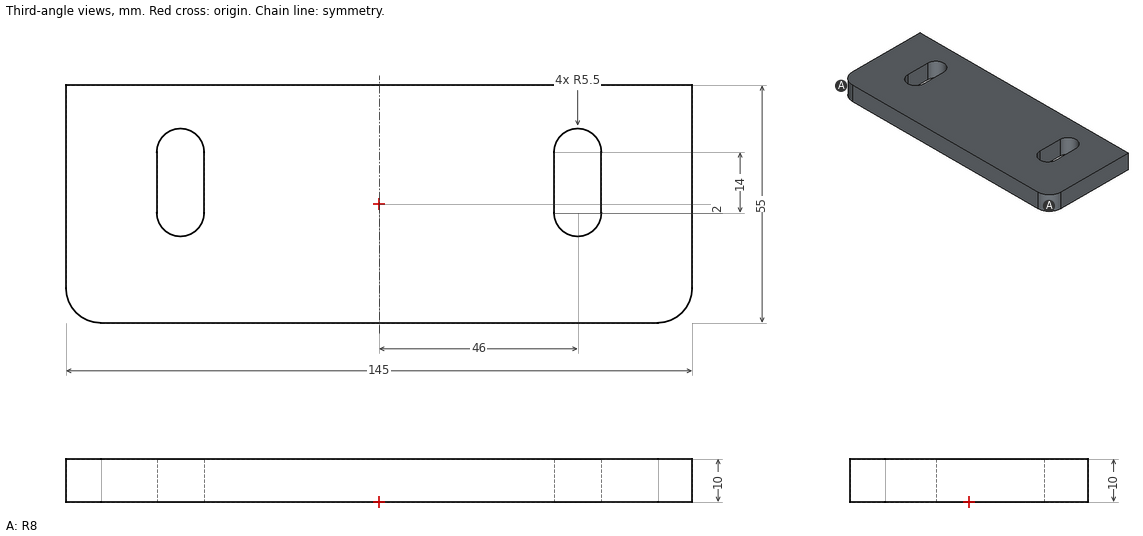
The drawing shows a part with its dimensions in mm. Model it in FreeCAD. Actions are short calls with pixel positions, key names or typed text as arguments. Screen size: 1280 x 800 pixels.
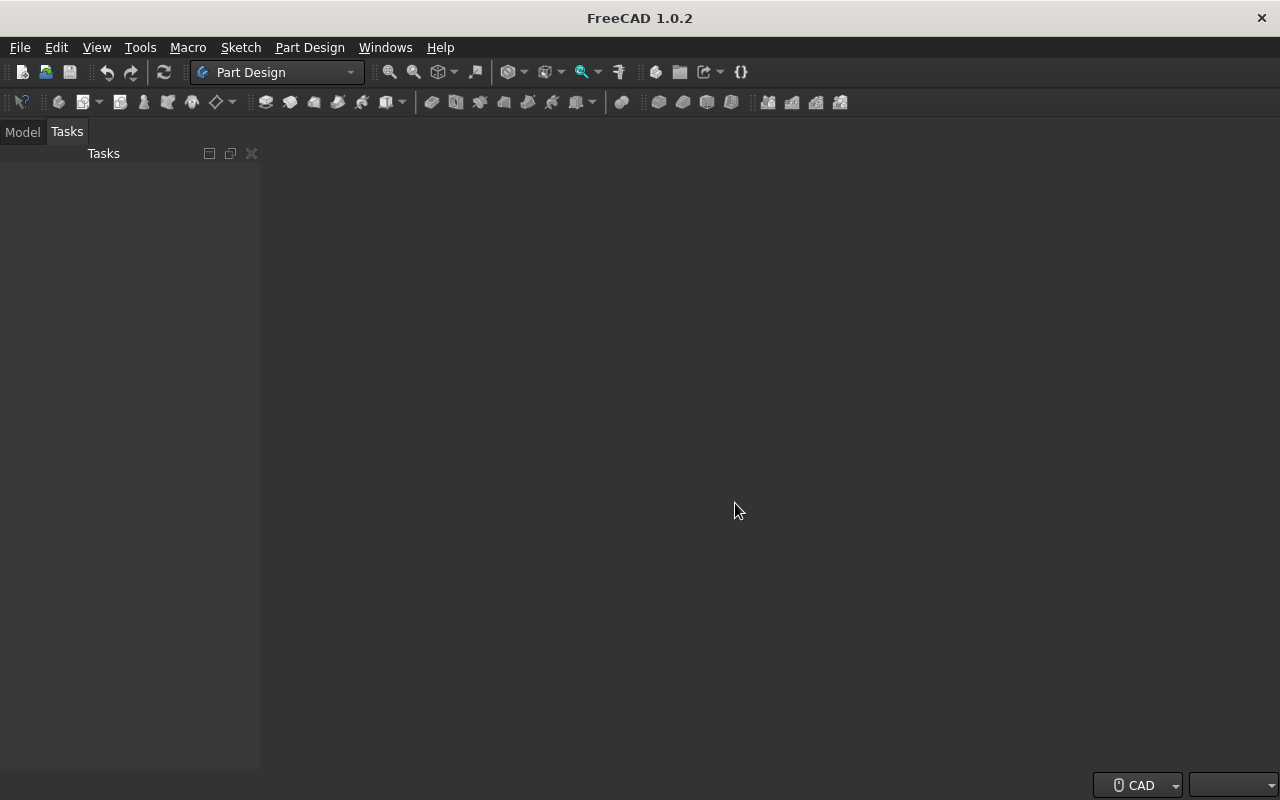
click(22, 72)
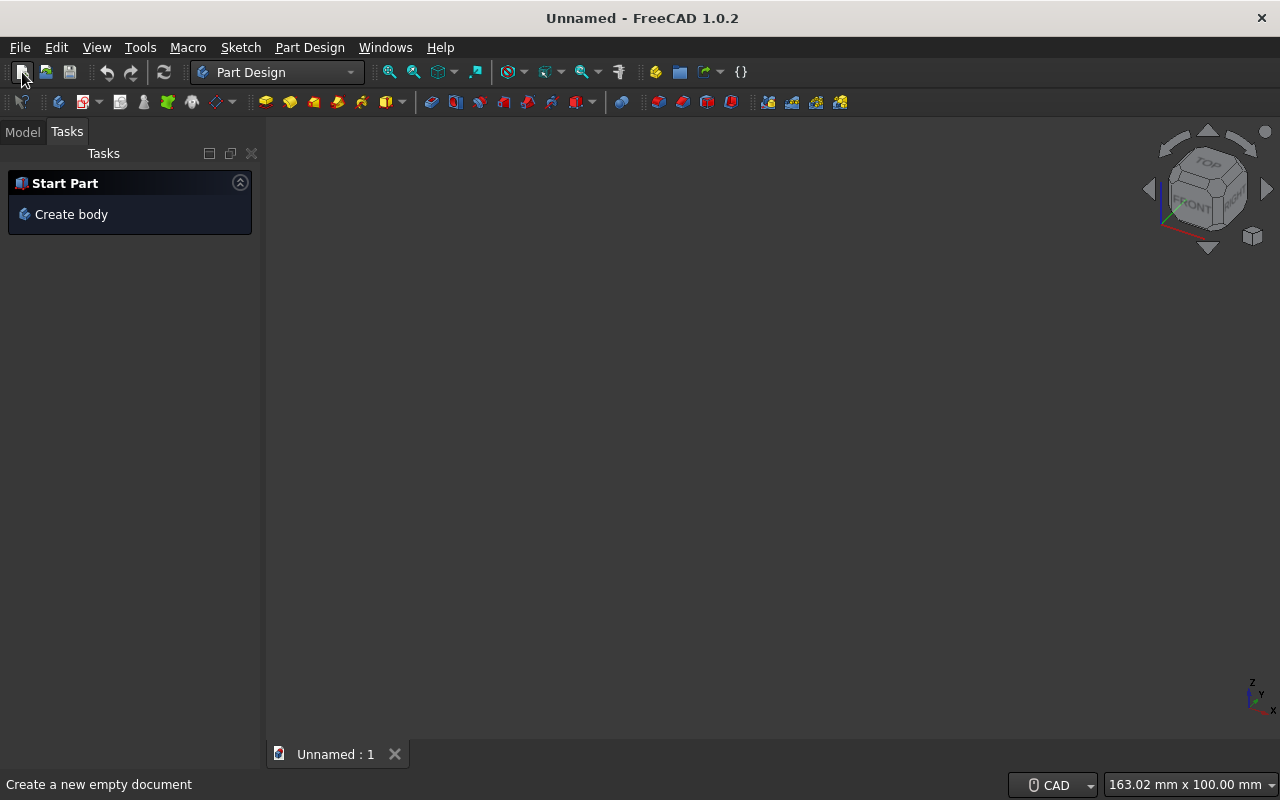
click(84, 102)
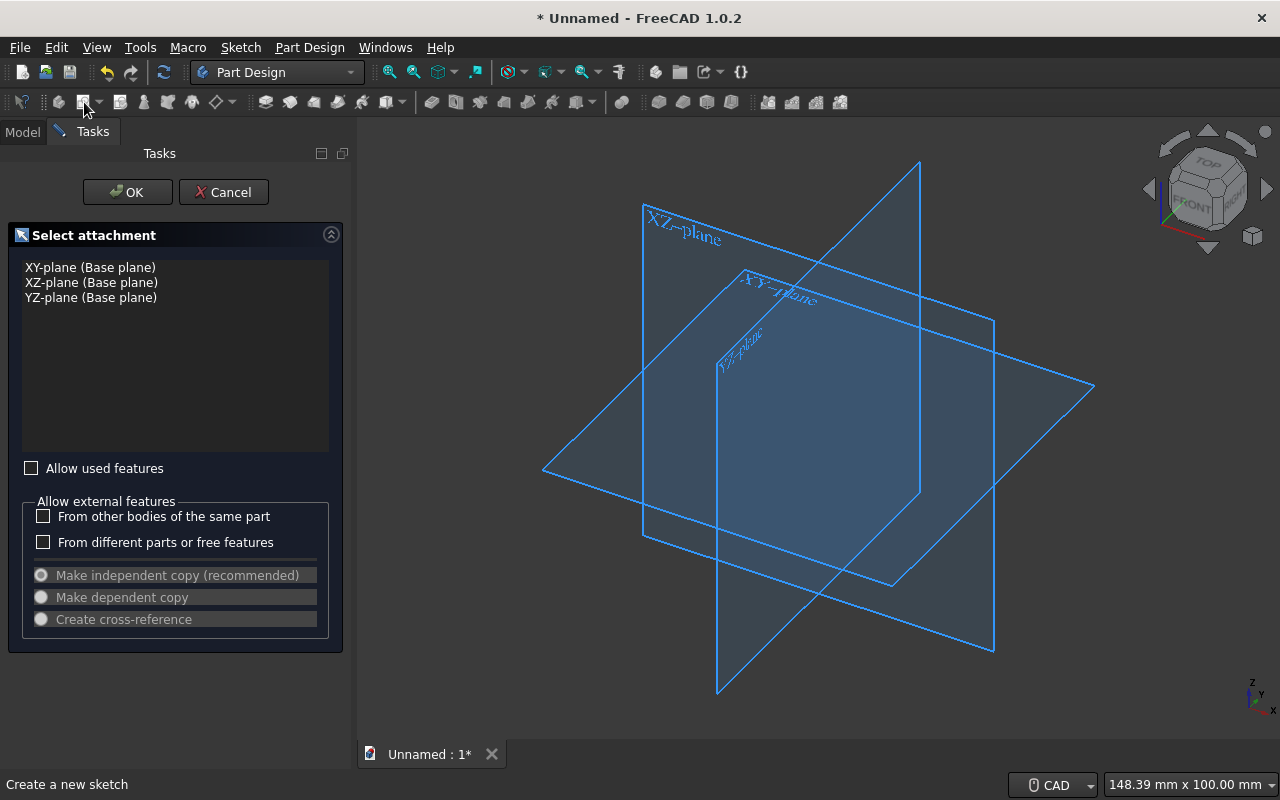
click(82, 268)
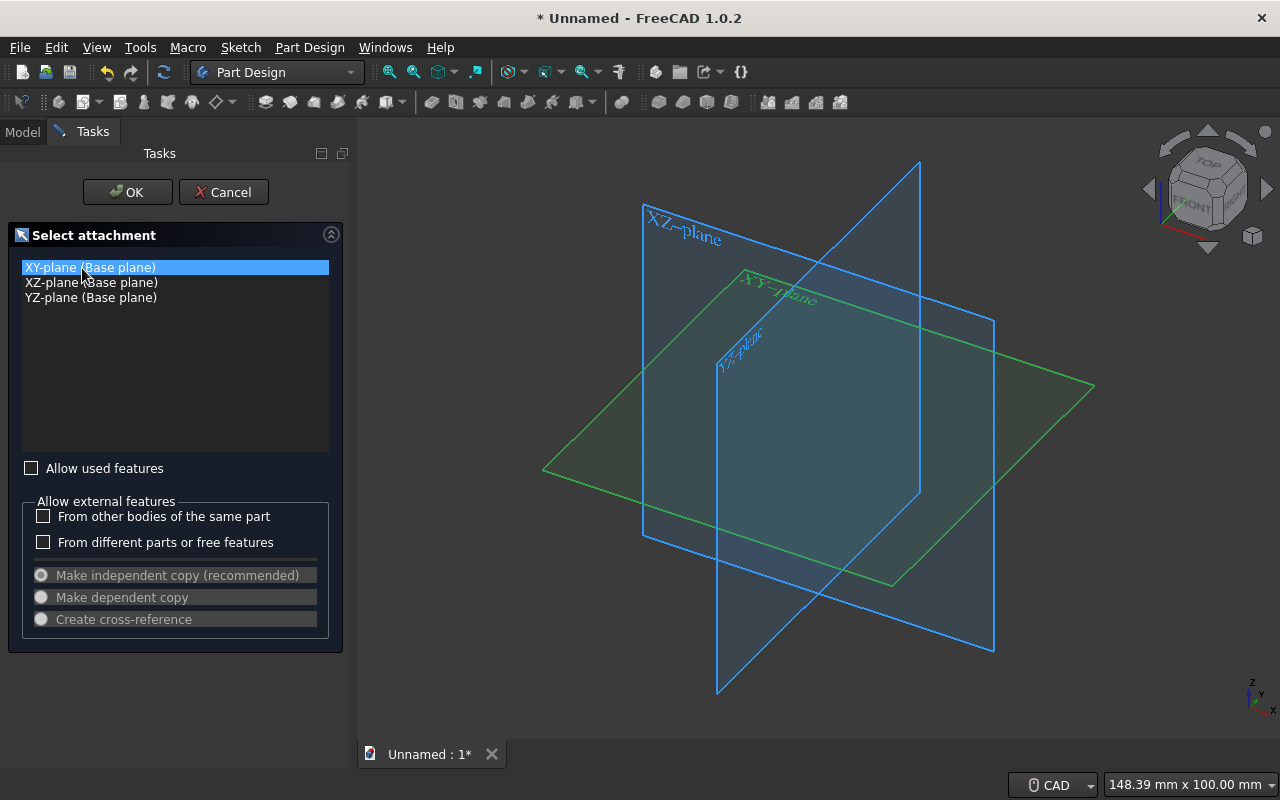
click(128, 192)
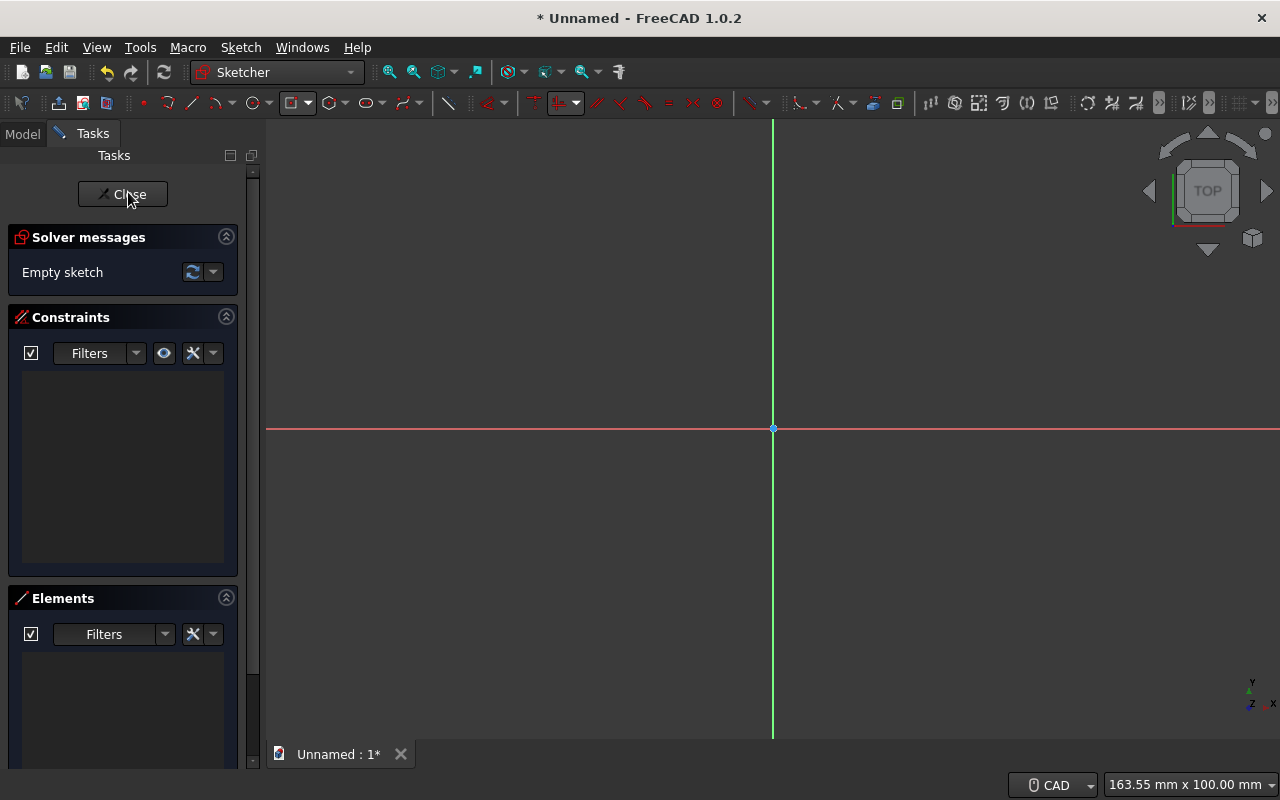
scroll(565, 429, down, 2)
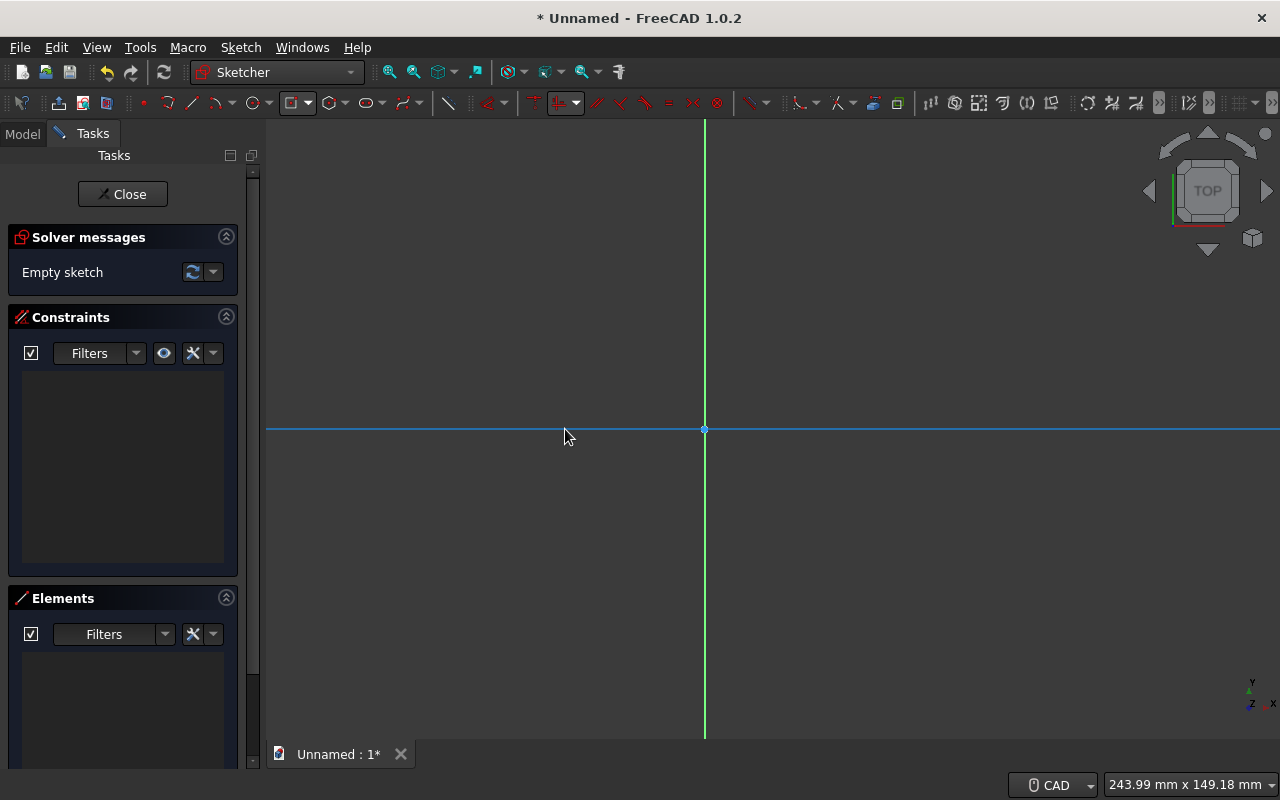
click(292, 104)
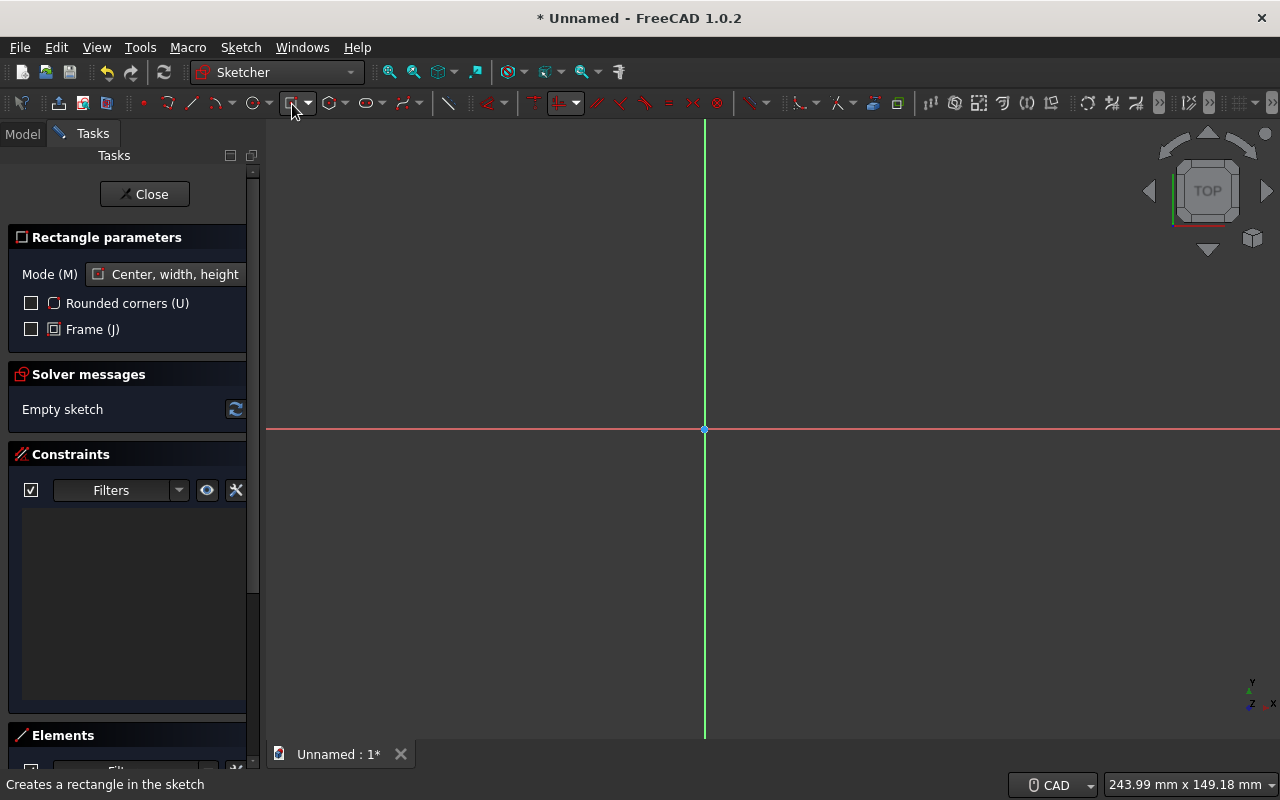
click(705, 429)
click(1006, 315)
key(Escape)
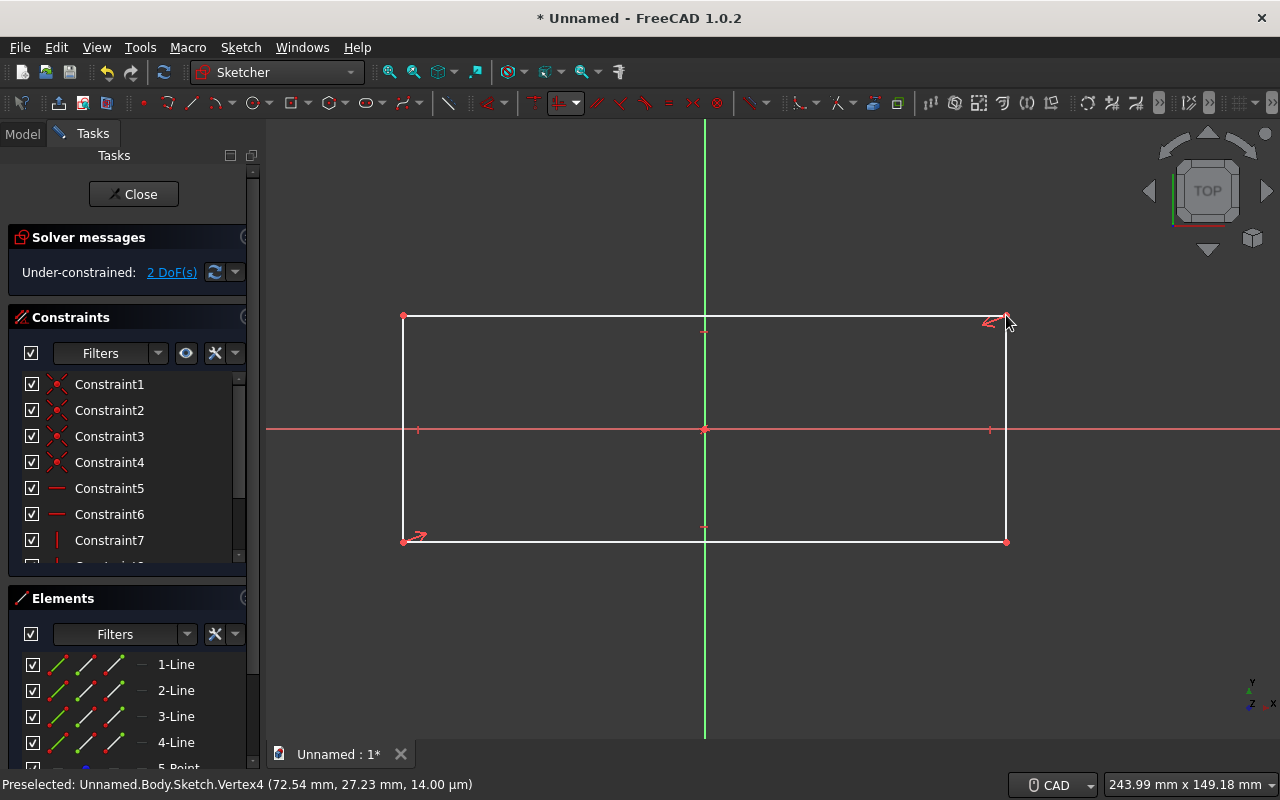
click(488, 104)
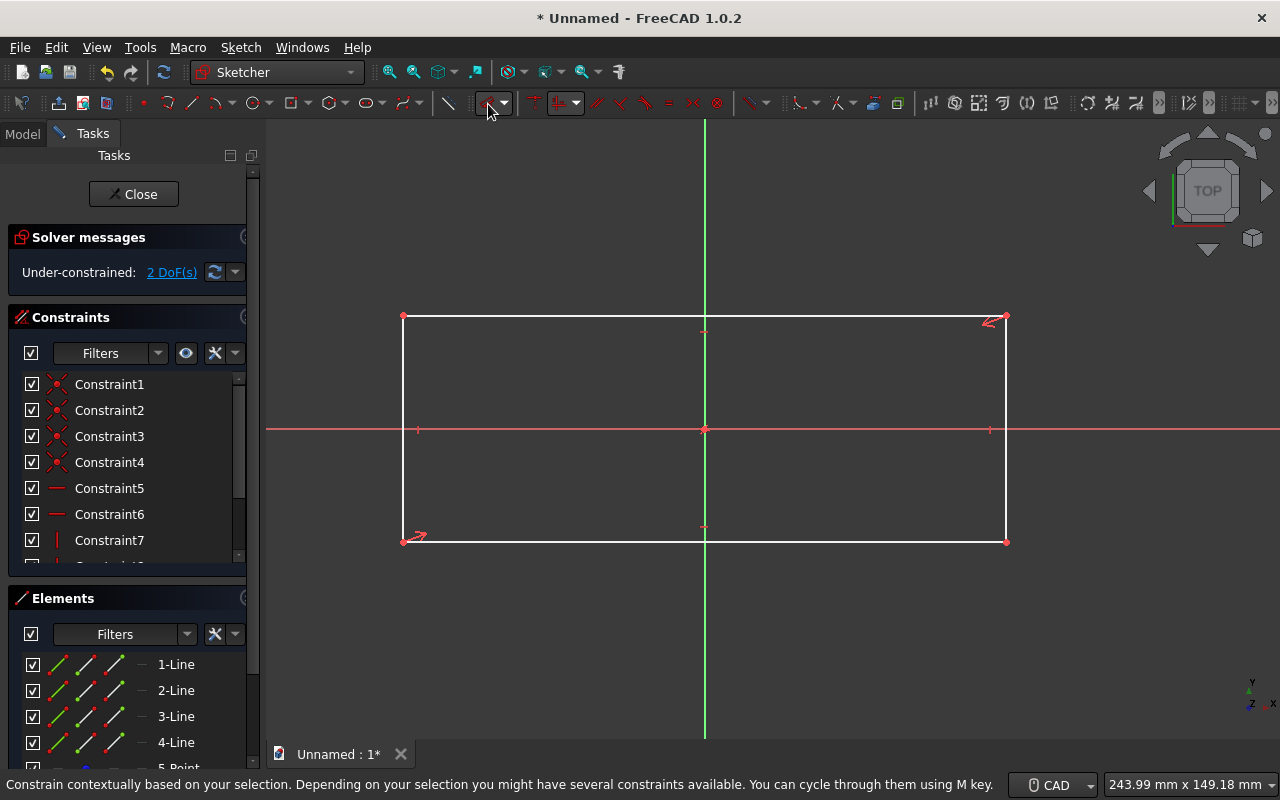
click(1006, 474)
click(1040, 377)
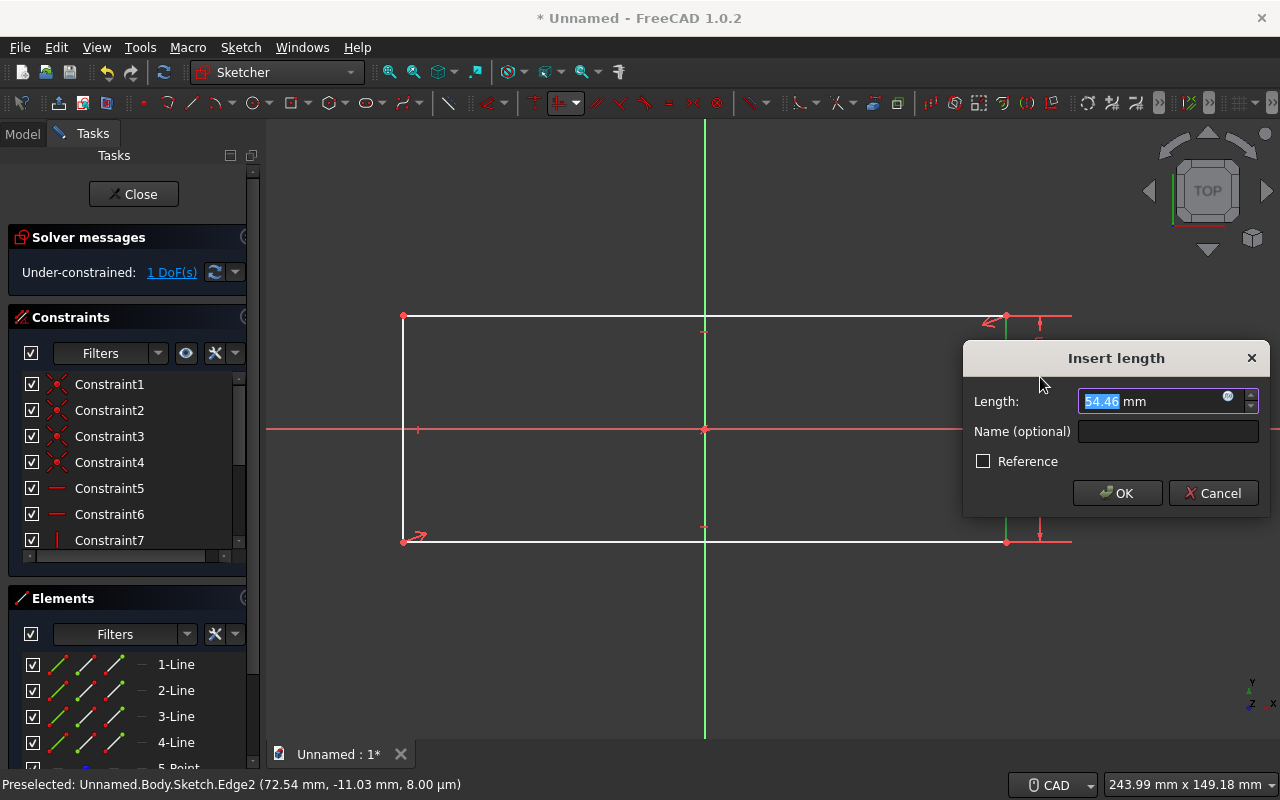
text(55)
key(Return)